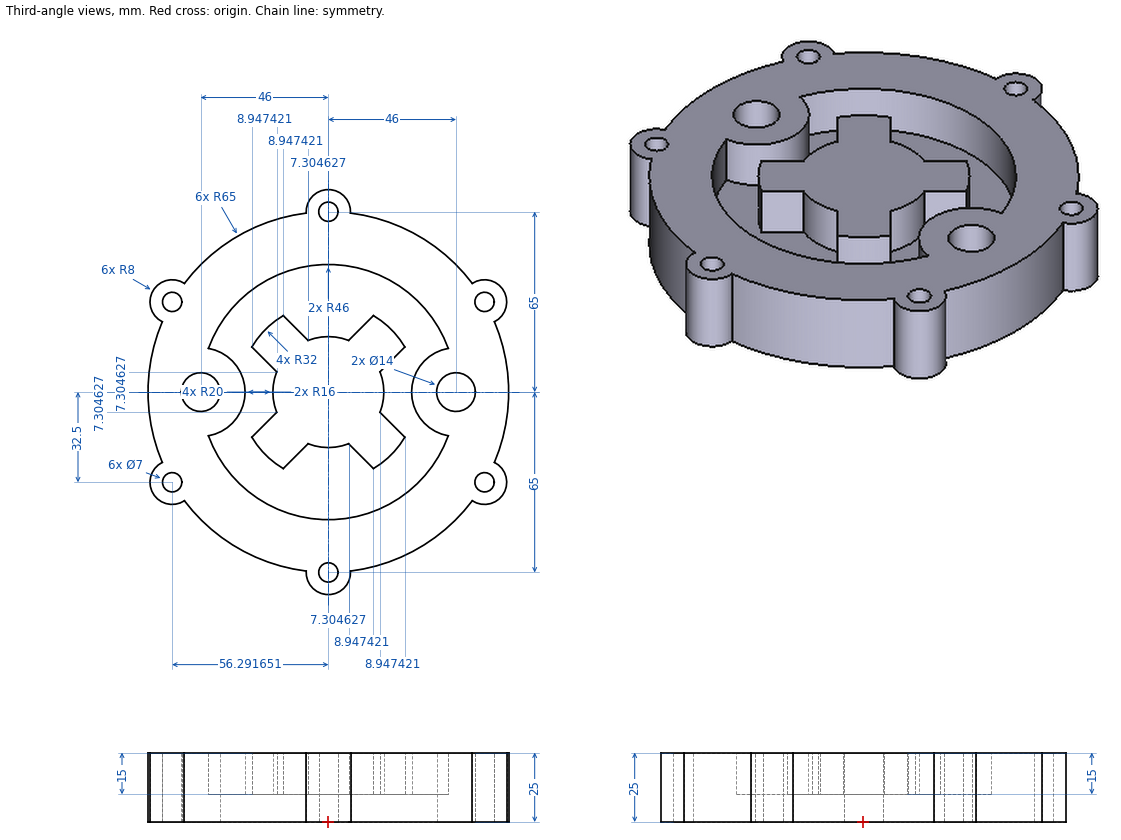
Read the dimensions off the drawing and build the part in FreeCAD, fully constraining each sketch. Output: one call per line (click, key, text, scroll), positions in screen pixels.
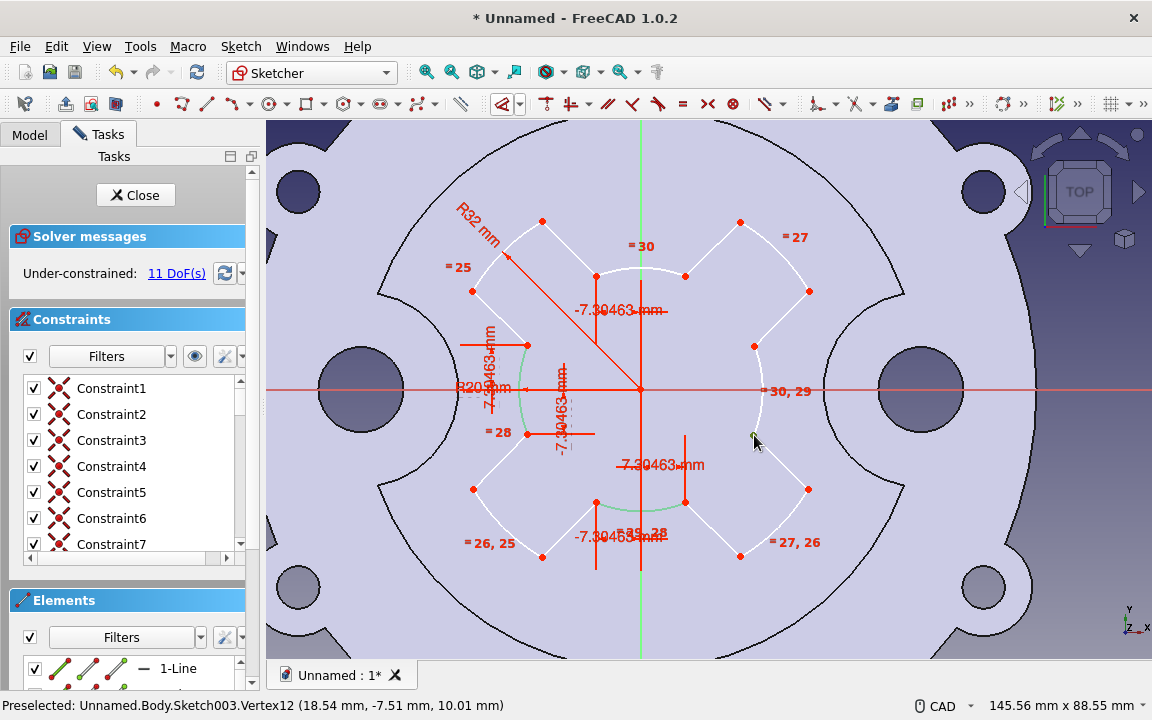
click(520, 104)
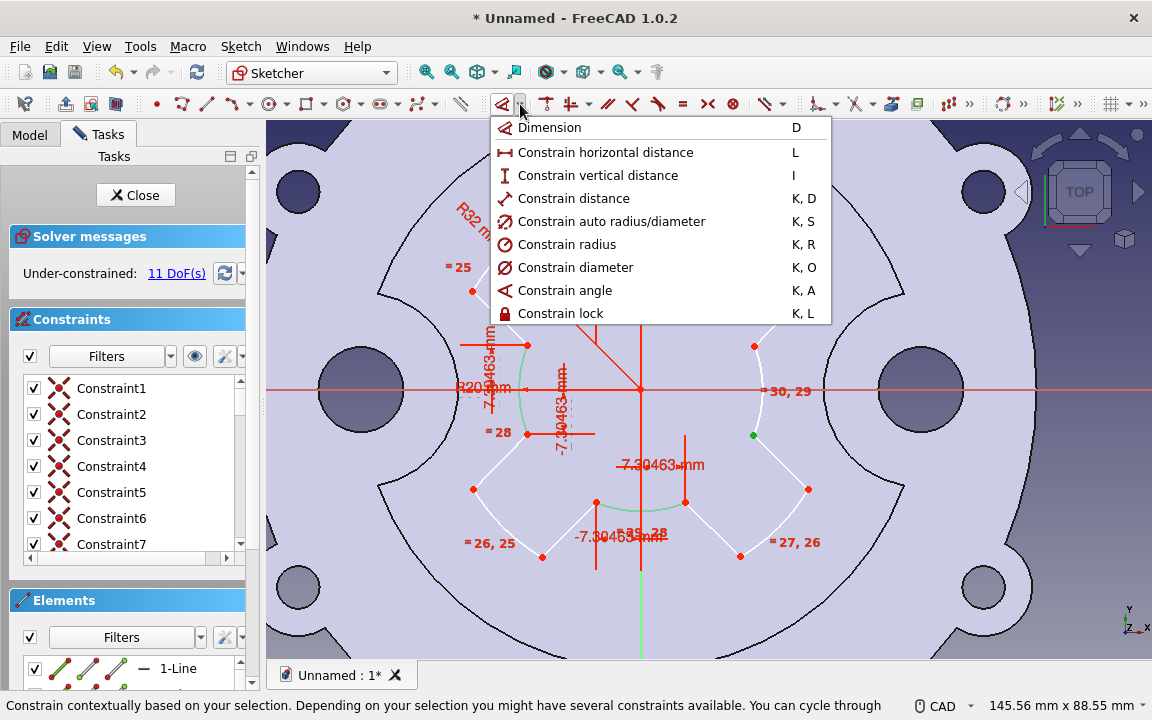
click(661, 176)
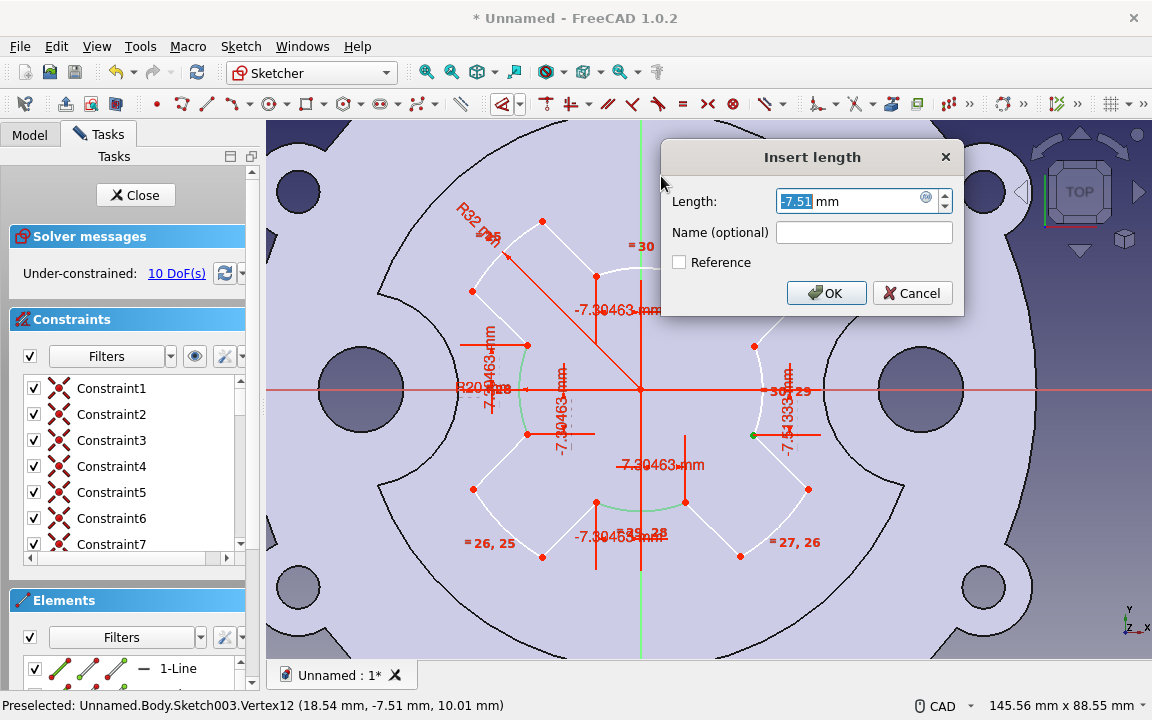
text(-7.304627)
key(Return)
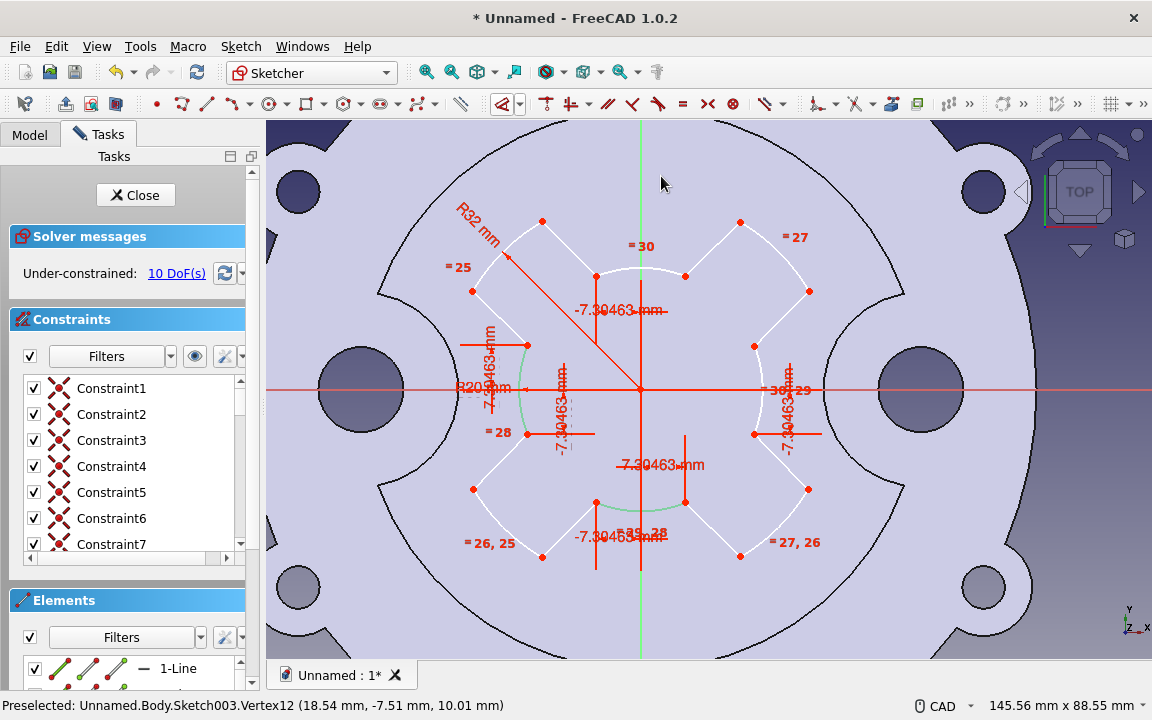
click(755, 346)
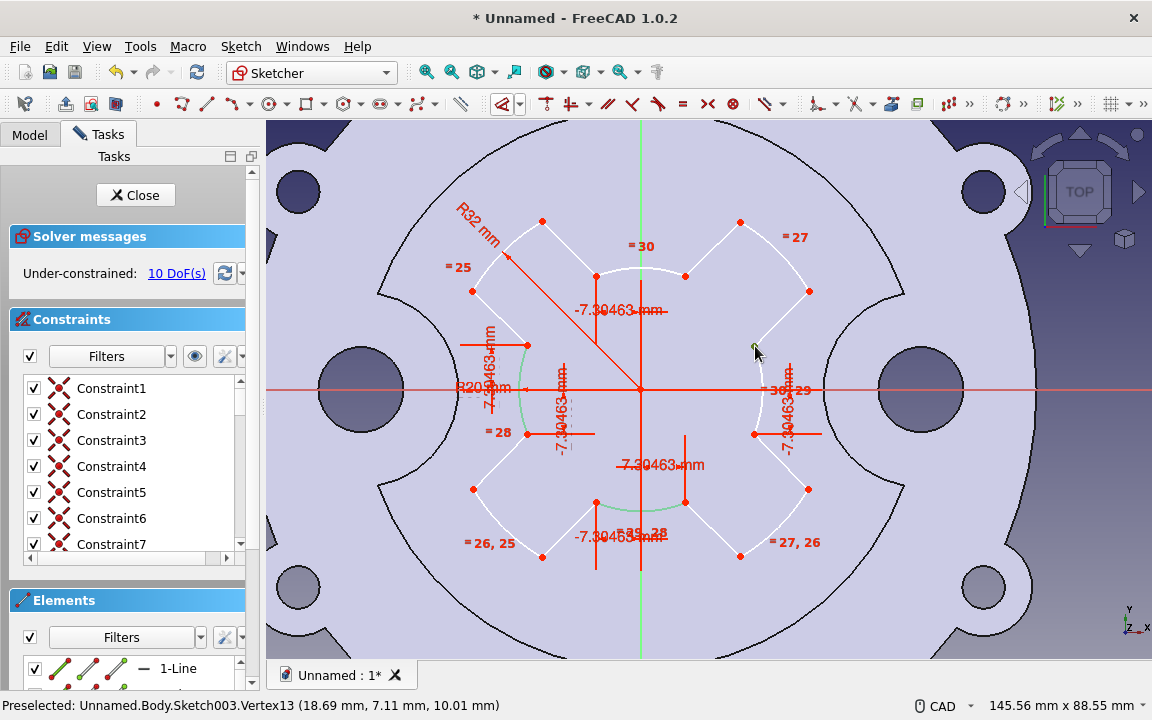
key(i)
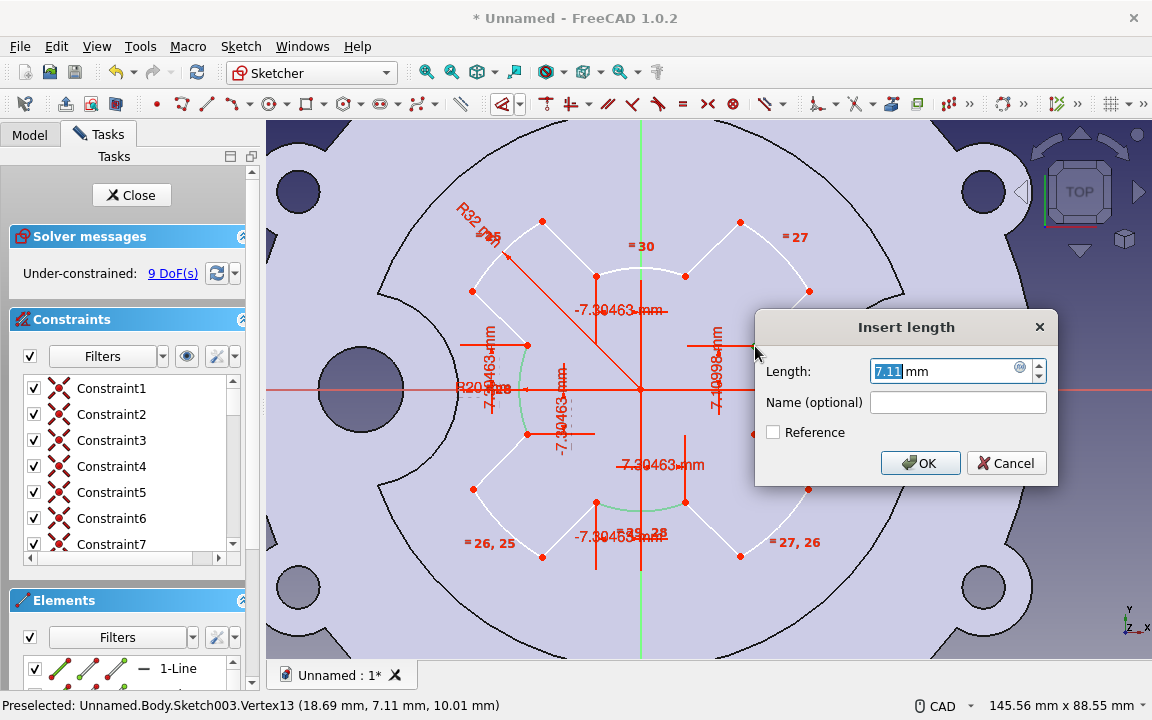
text(7.304627)
key(Return)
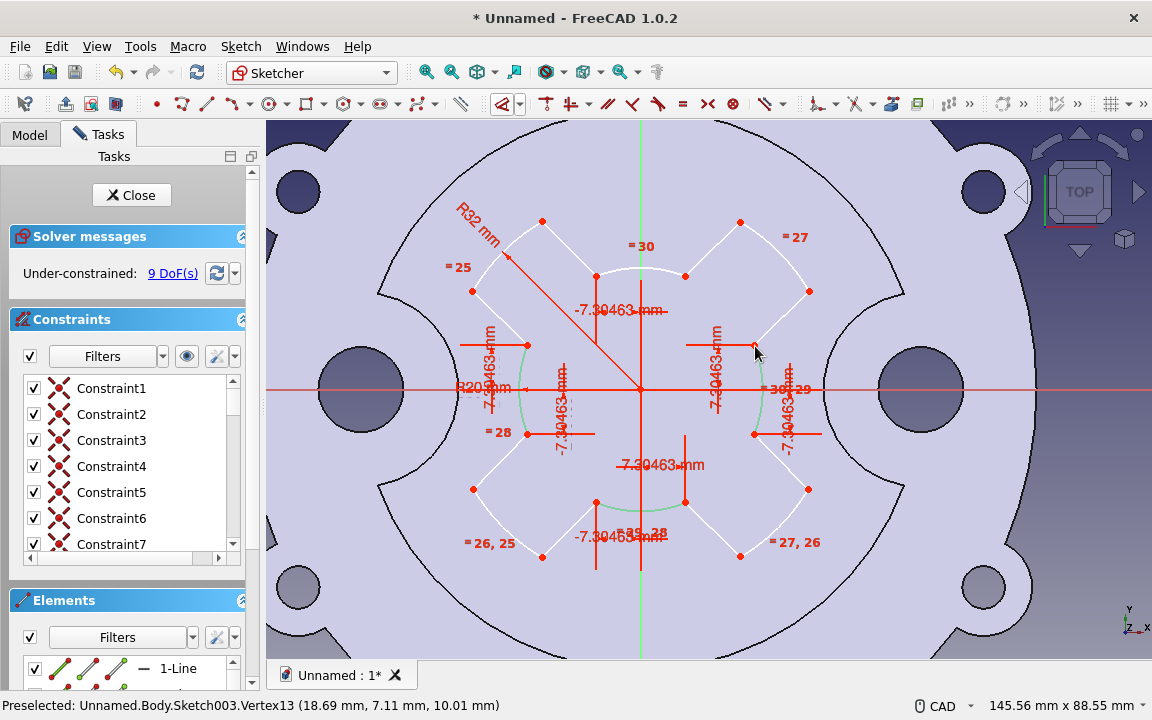
click(685, 276)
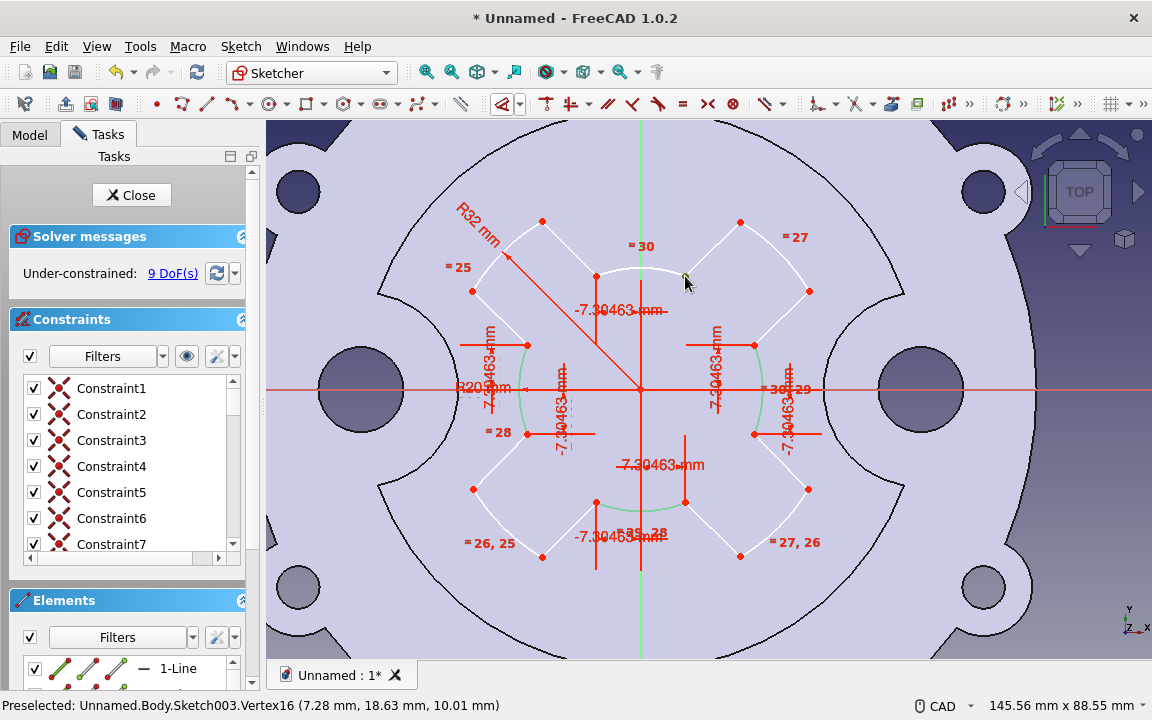
key(l)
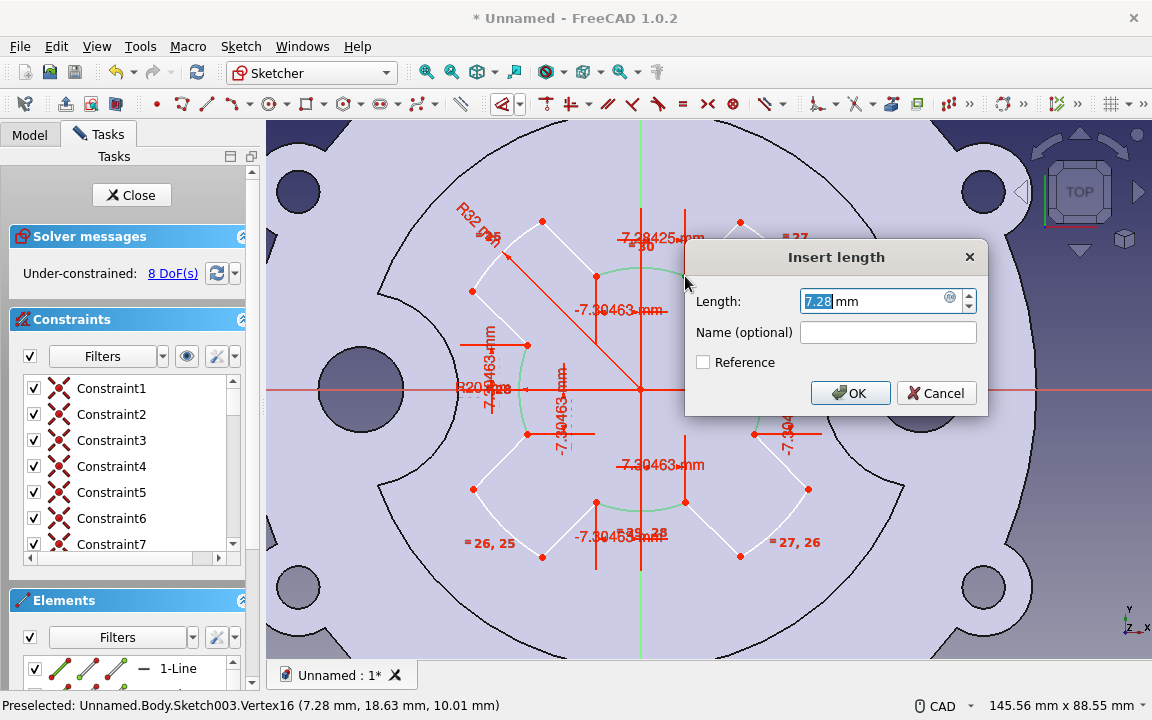
text(7.304627)
key(Return)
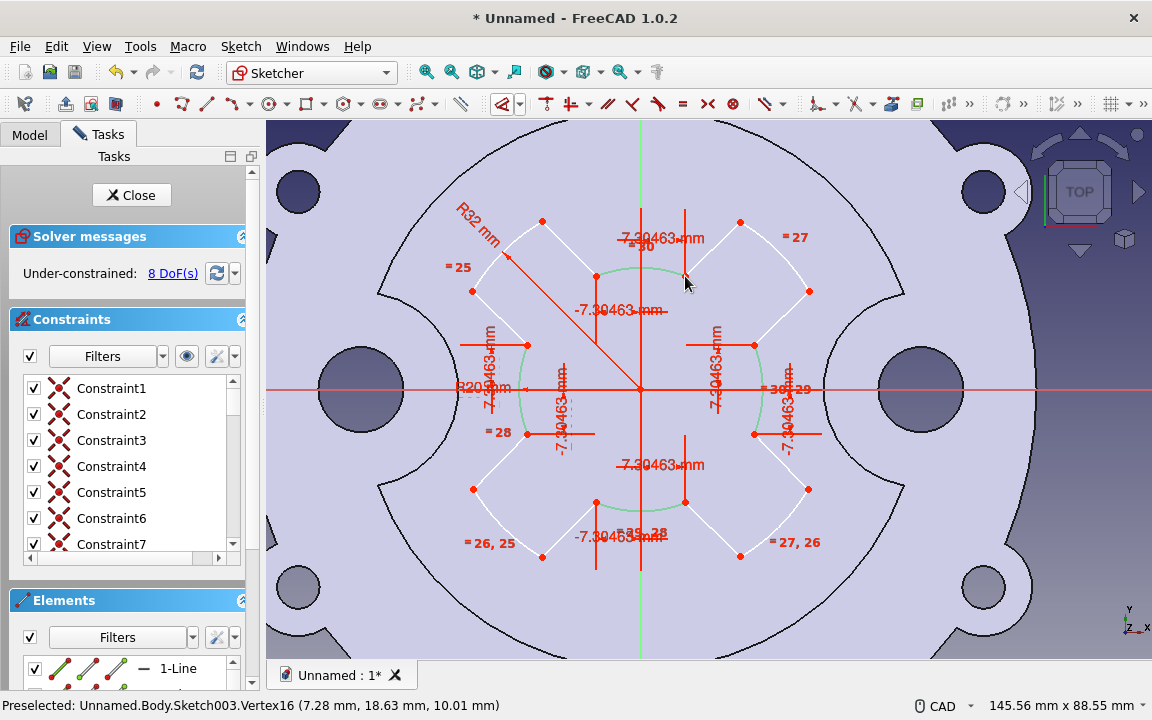
click(580, 260)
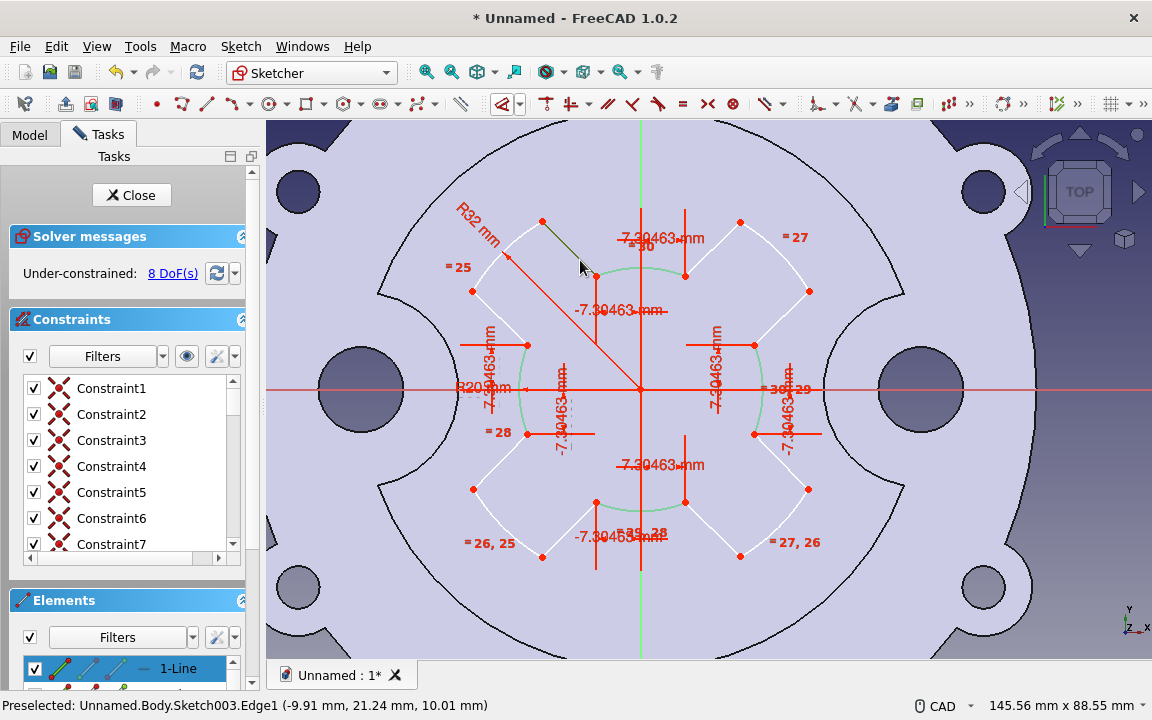
key(l)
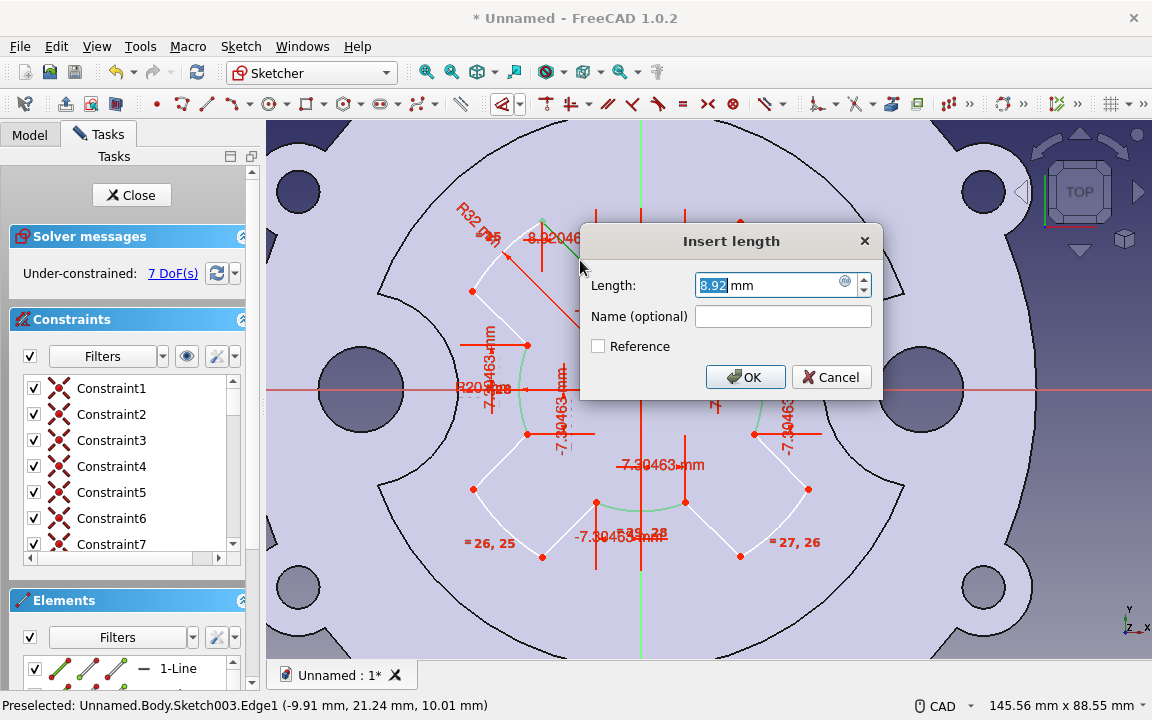
text(8.947421)
key(Return)